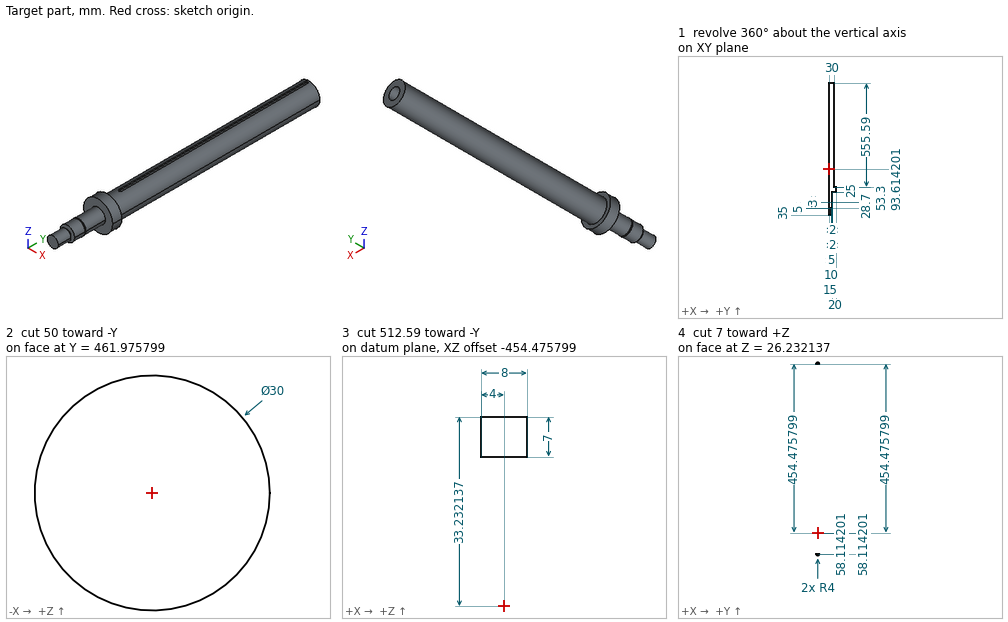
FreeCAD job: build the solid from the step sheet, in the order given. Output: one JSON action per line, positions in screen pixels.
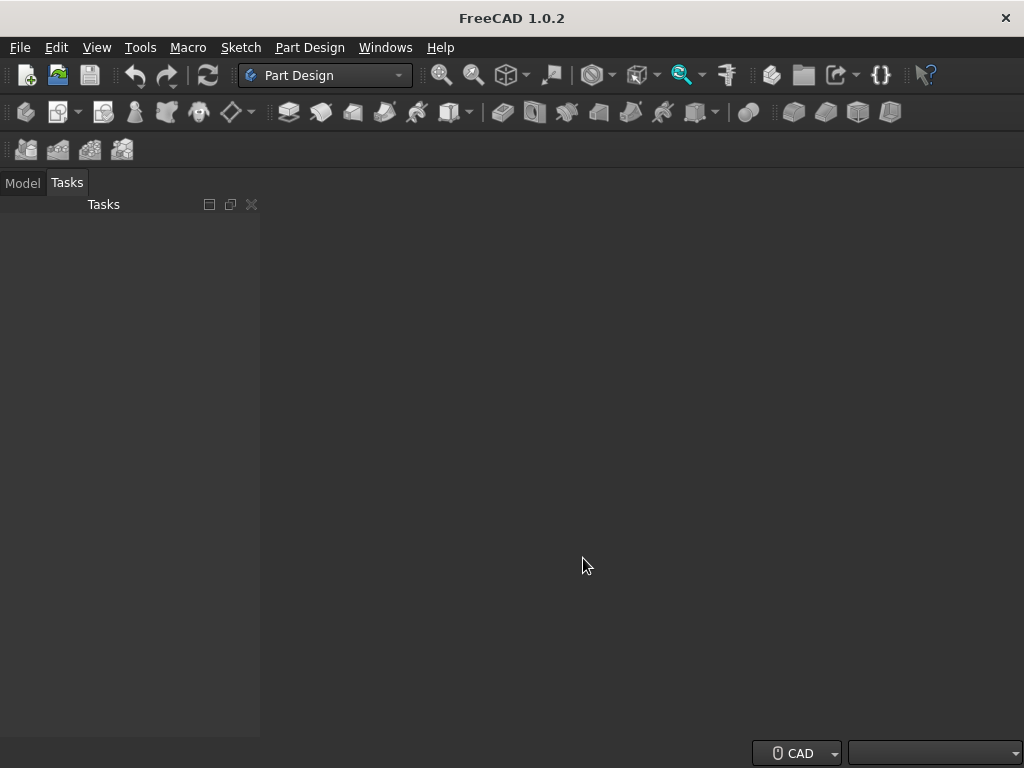
{"action": "key", "text": "ctrl+n"}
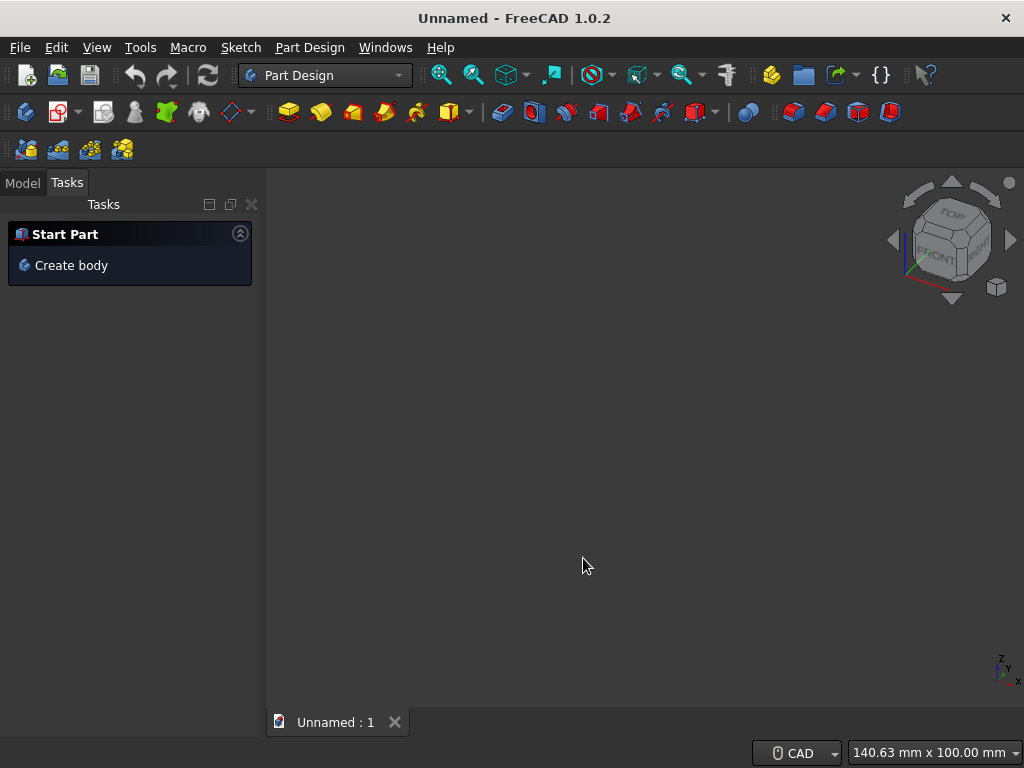
{"action": "left_click", "coordinate": [58, 112]}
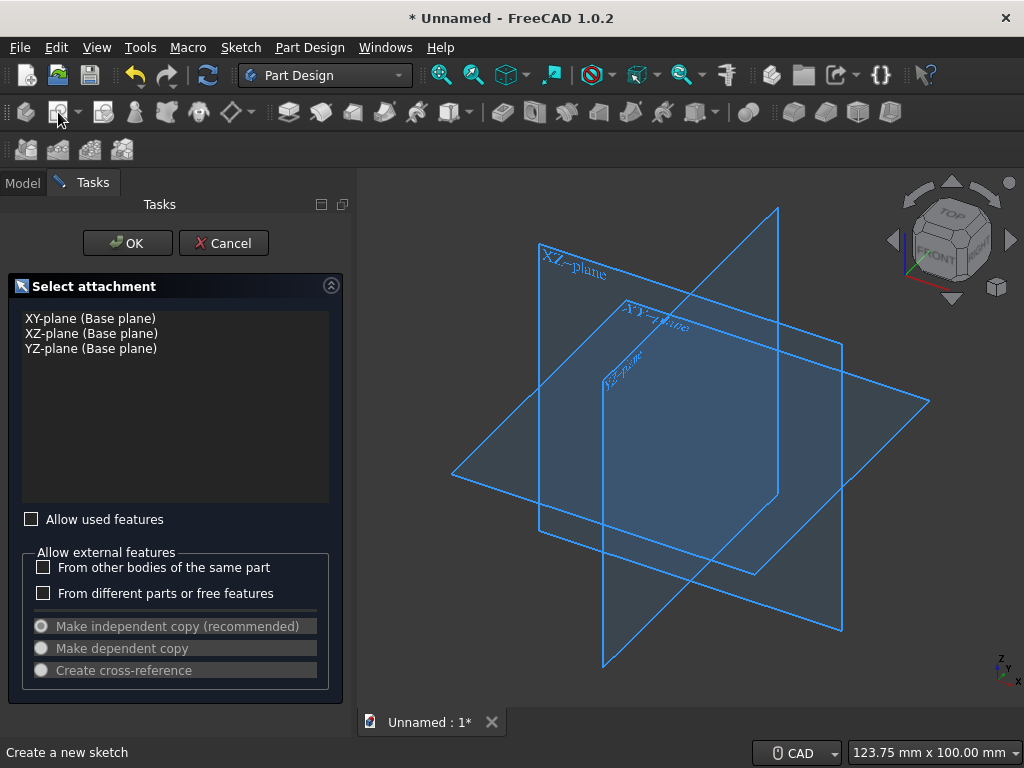
{"action": "left_click", "coordinate": [82, 318]}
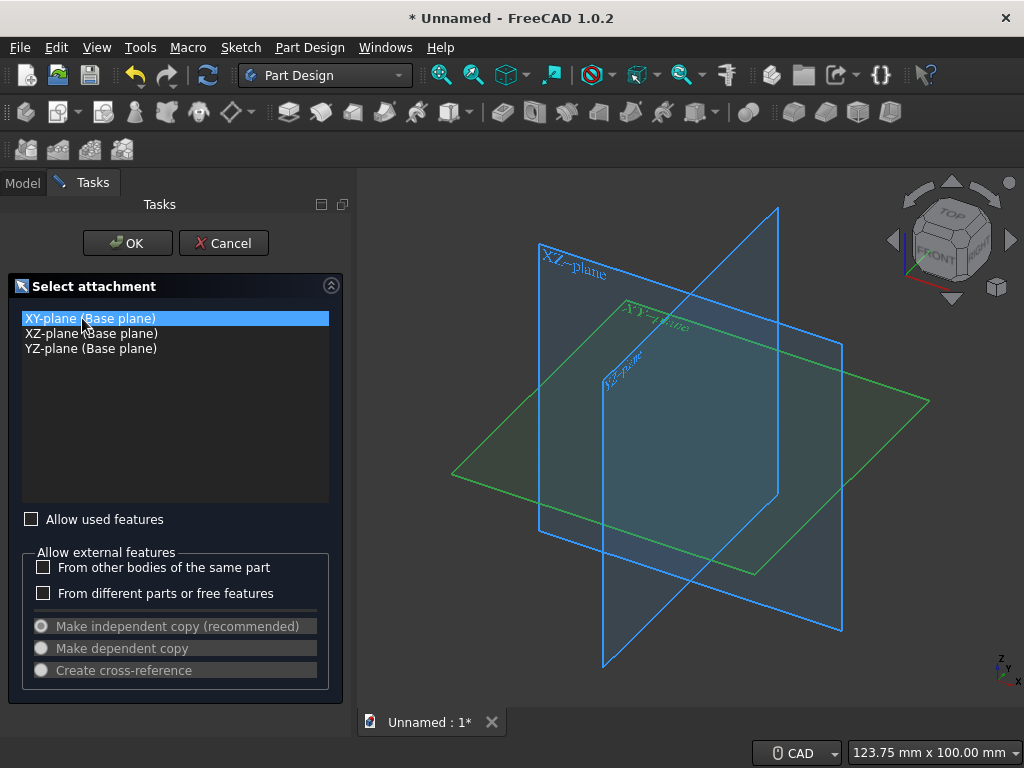
{"action": "left_click", "coordinate": [128, 243]}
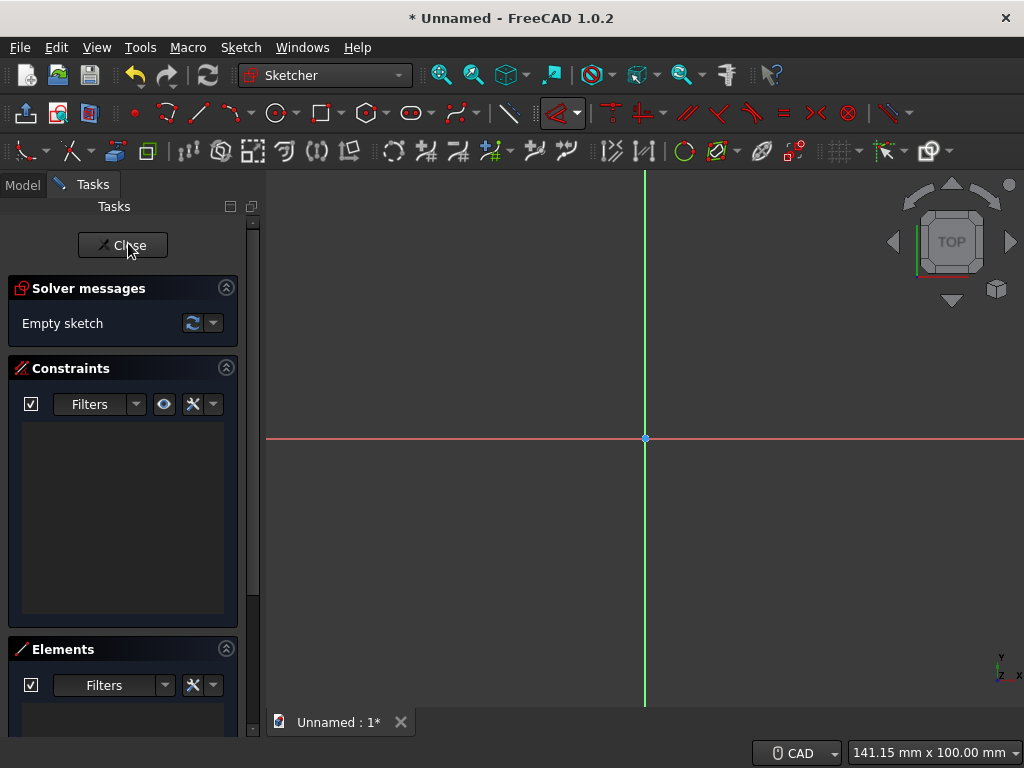
{"action": "scroll", "coordinate": [559, 497], "scroll_direction": "down", "scroll_amount": 12}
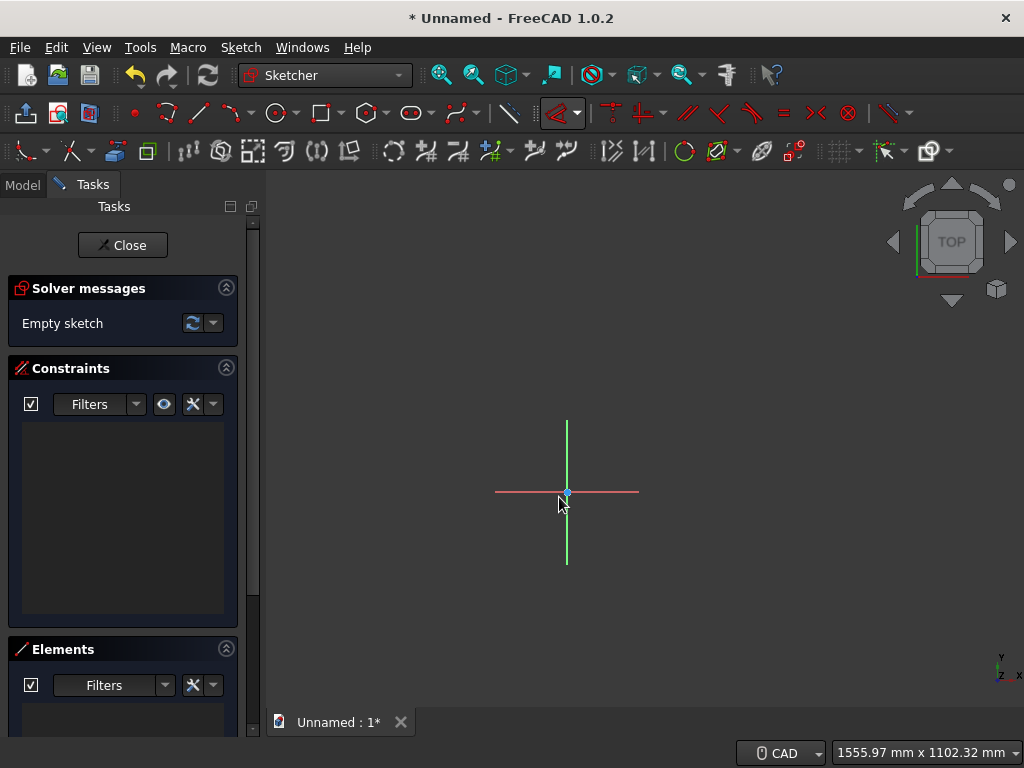
{"action": "key", "text": "g m"}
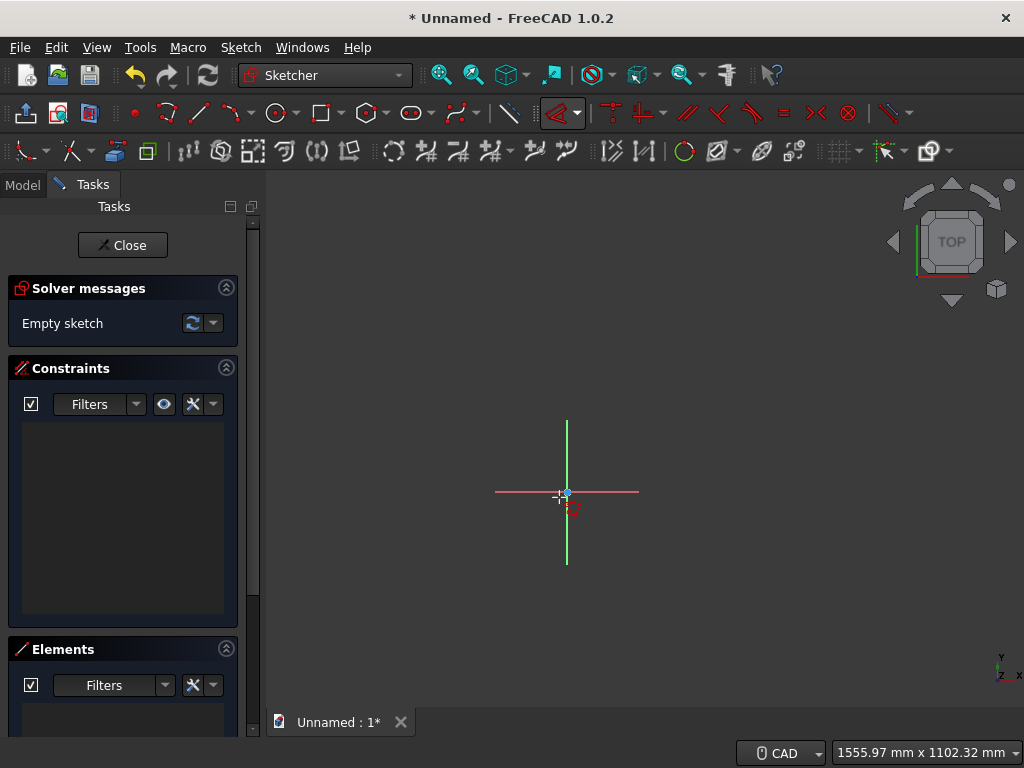
{"action": "left_click", "coordinate": [582, 538]}
{"action": "left_click", "coordinate": [582, 267]}
{"action": "left_click", "coordinate": [567, 267]}
{"action": "left_click", "coordinate": [576, 611]}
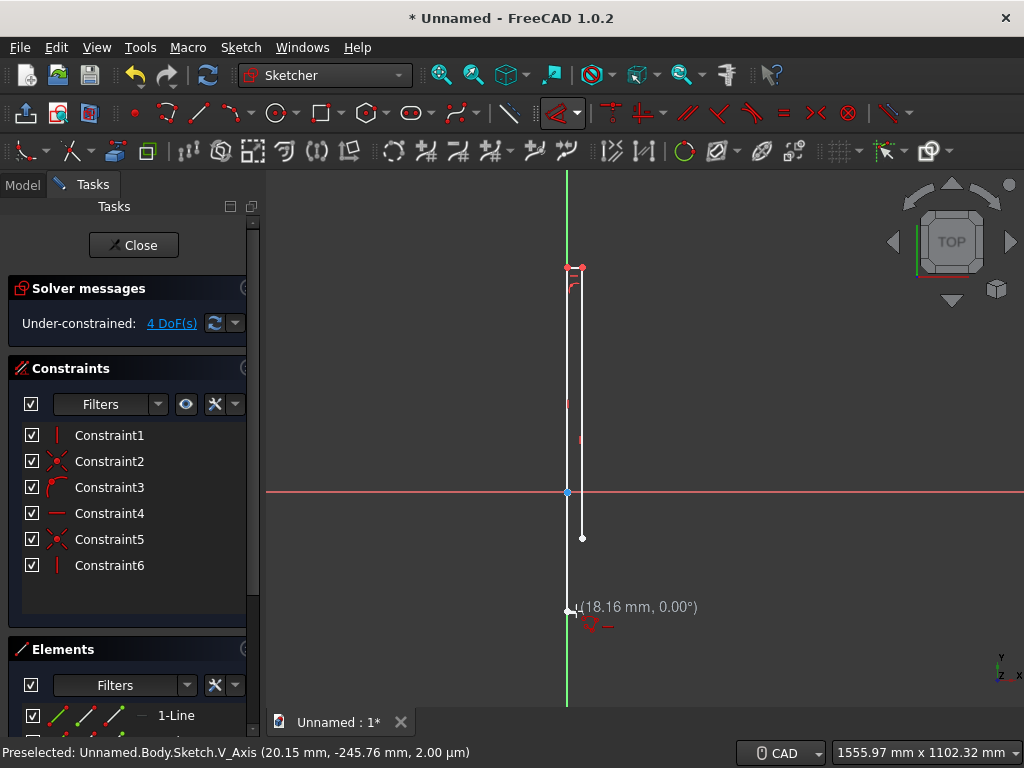
{"action": "scroll", "coordinate": [574, 611], "scroll_direction": "up", "scroll_amount": 4}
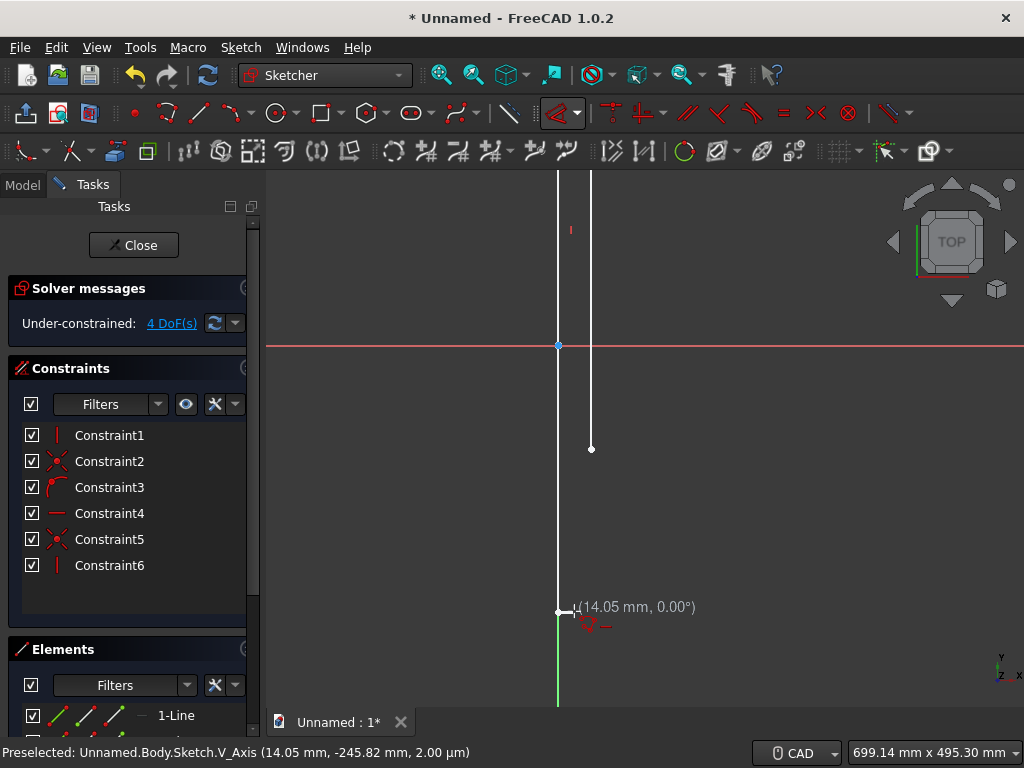
{"action": "left_click", "coordinate": [575, 610]}
{"action": "left_click", "coordinate": [575, 572]}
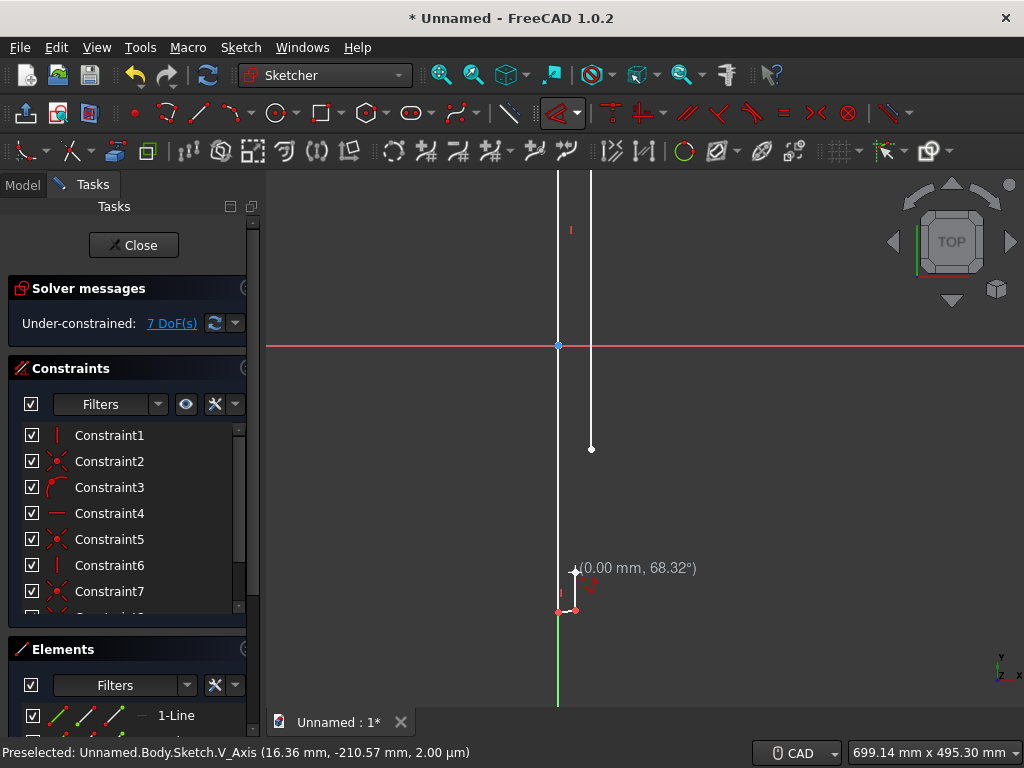
{"action": "scroll", "coordinate": [569, 572], "scroll_direction": "up", "scroll_amount": 6}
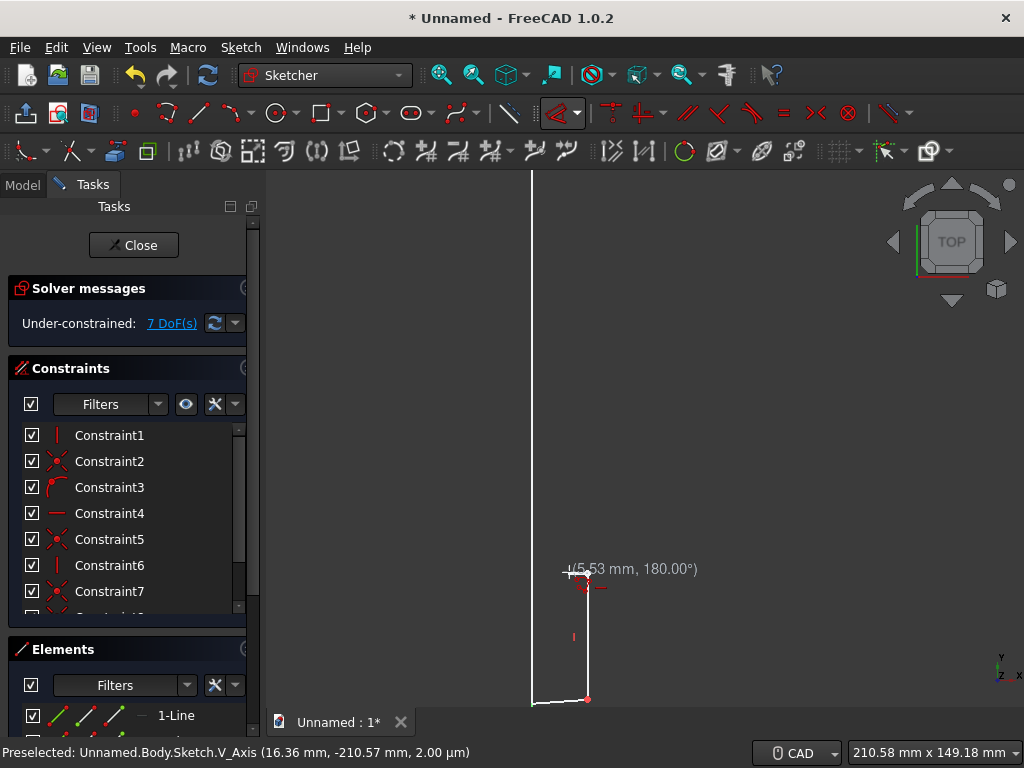
{"action": "left_click", "coordinate": [568, 570]}
{"action": "left_click", "coordinate": [568, 552]}
{"action": "left_click", "coordinate": [604, 552]}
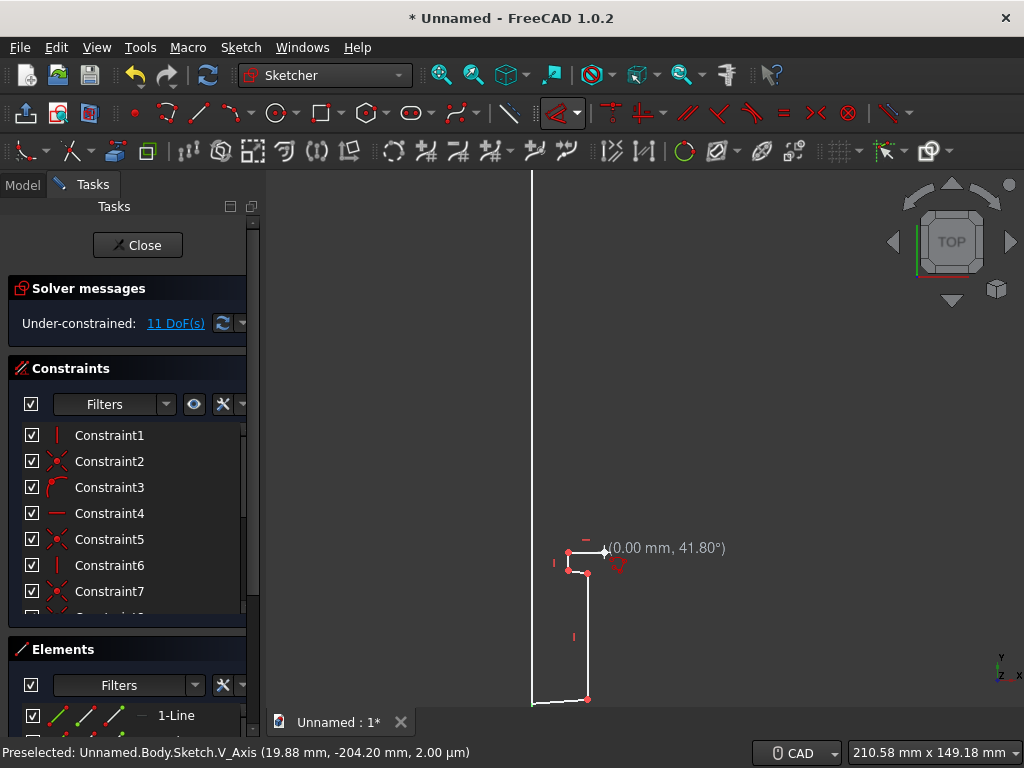
{"action": "scroll", "coordinate": [572, 597], "scroll_direction": "down", "scroll_amount": 10}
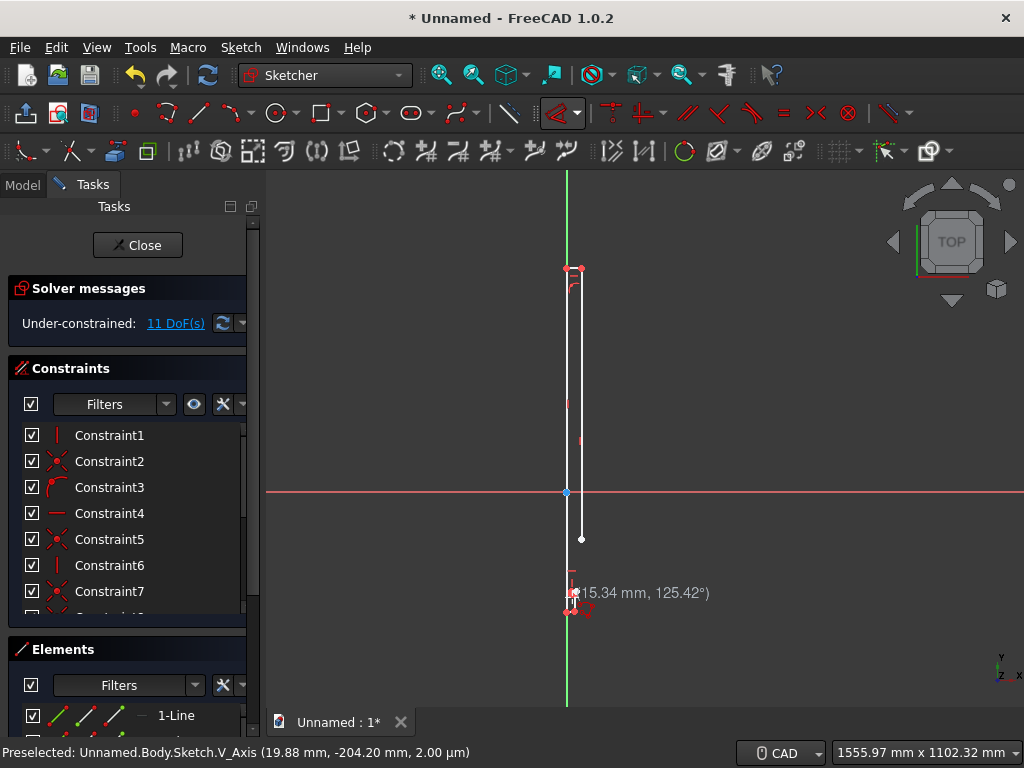
{"action": "scroll", "coordinate": [577, 578], "scroll_direction": "up", "scroll_amount": 3}